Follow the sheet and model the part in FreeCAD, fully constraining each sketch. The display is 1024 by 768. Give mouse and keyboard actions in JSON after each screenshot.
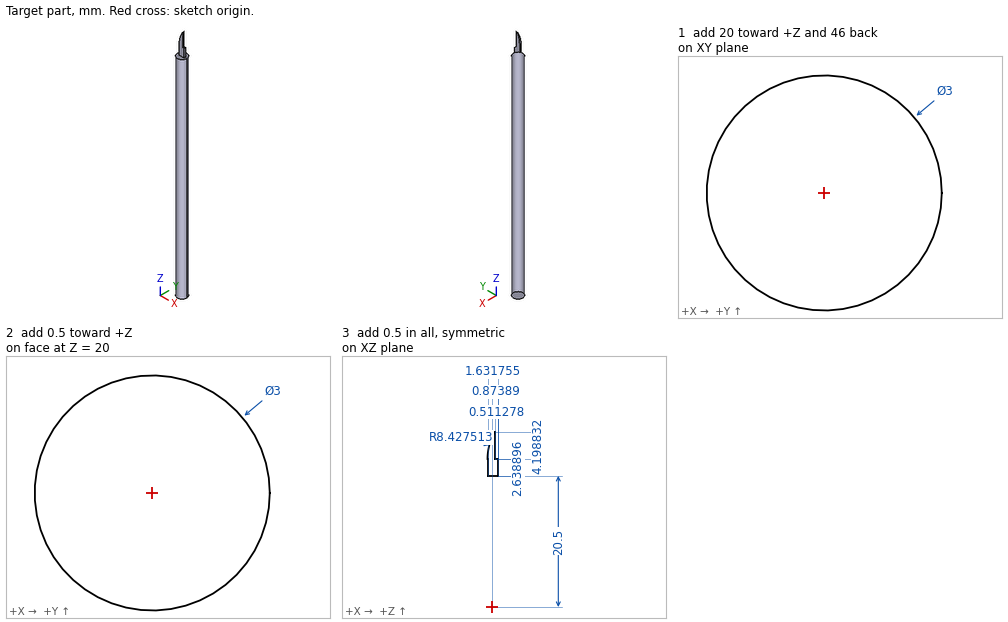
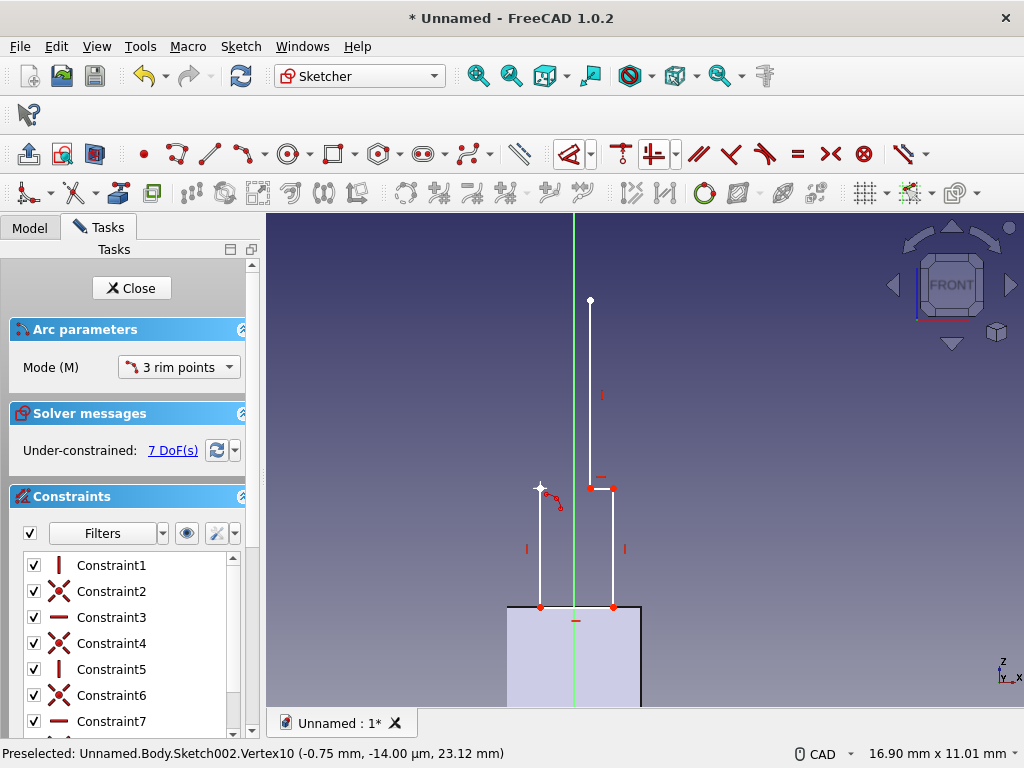
{"action": "left_click", "coordinate": [540, 489]}
{"action": "left_click", "coordinate": [590, 301]}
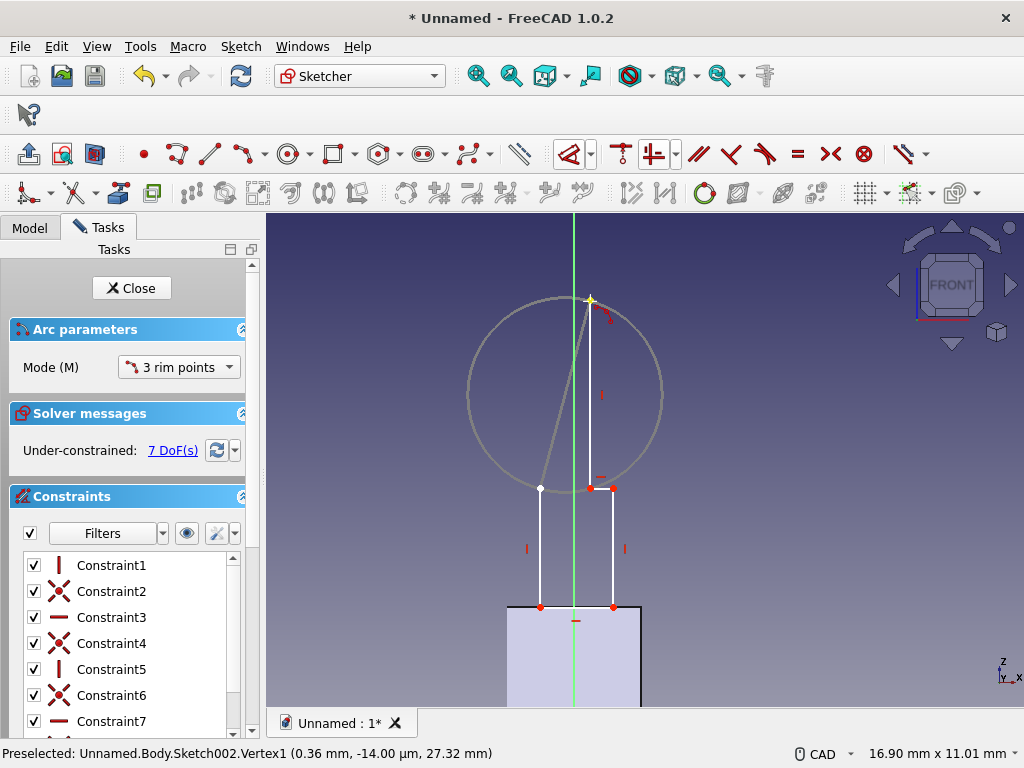
{"action": "scroll", "coordinate": [553, 391], "scroll_direction": "up", "scroll_amount": 2}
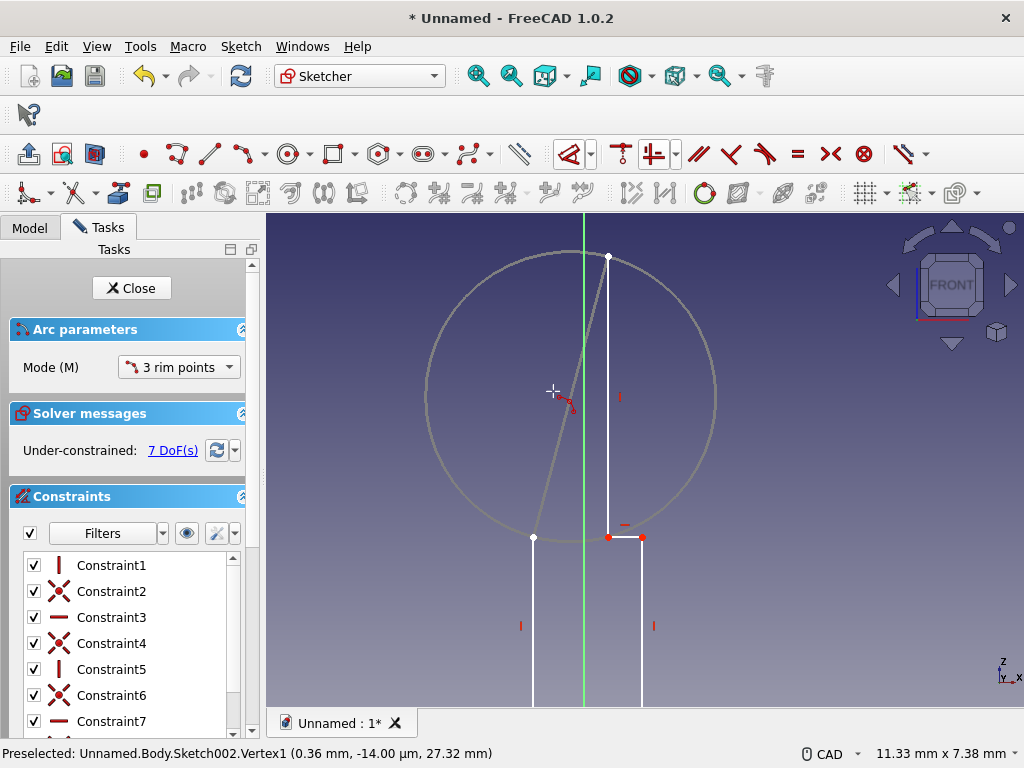
{"action": "left_click", "coordinate": [552, 391]}
{"action": "key", "text": "Escape"}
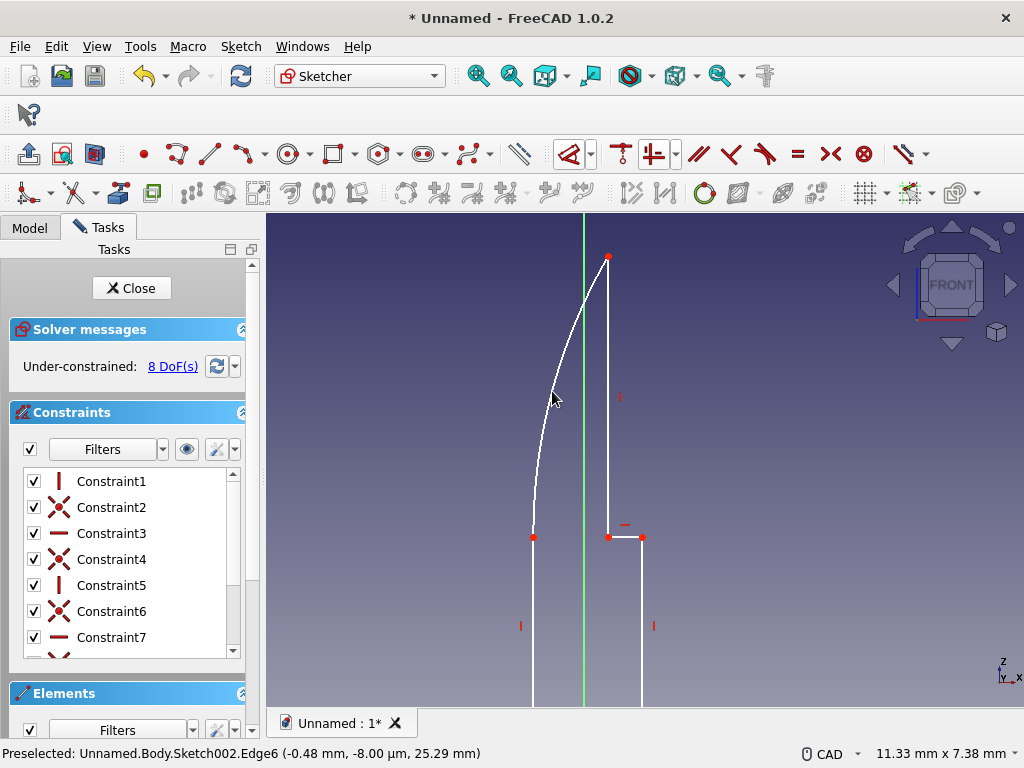
{"action": "left_click", "coordinate": [533, 661]}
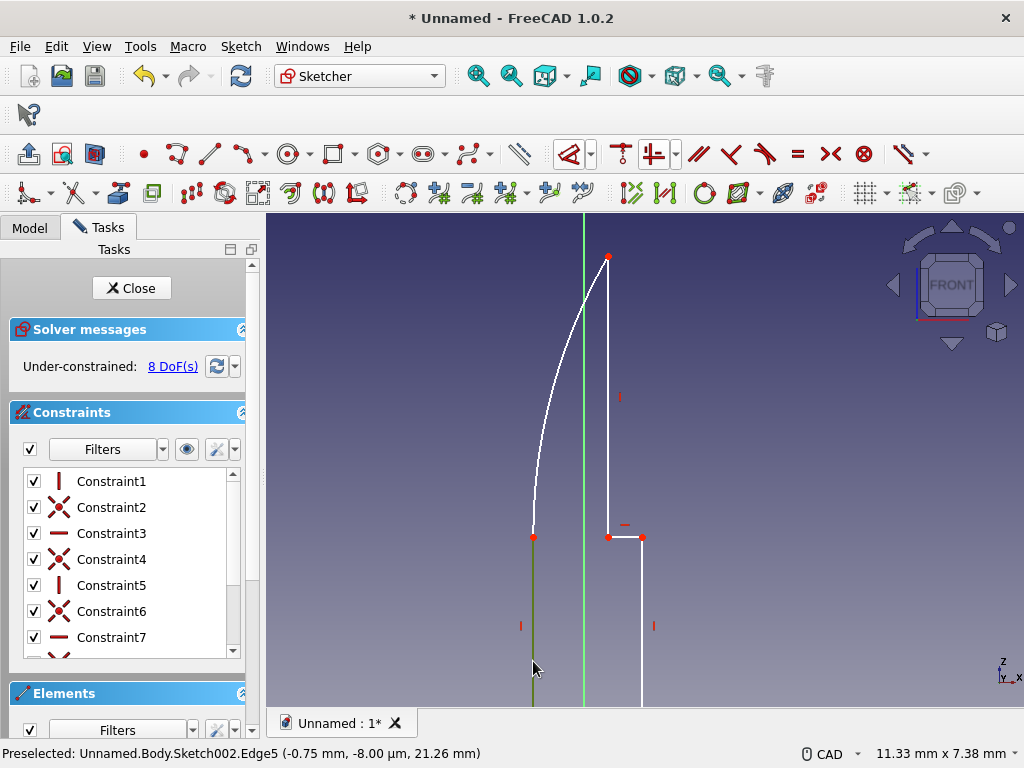
{"action": "left_click", "coordinate": [570, 336]}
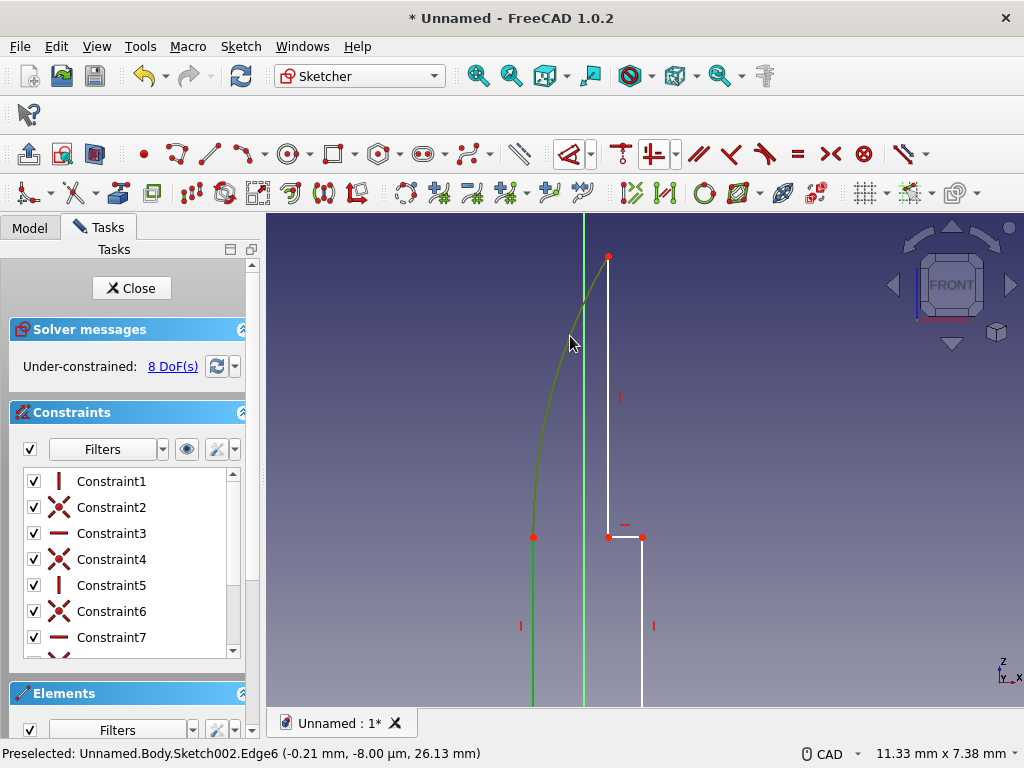
{"action": "left_click", "coordinate": [765, 154]}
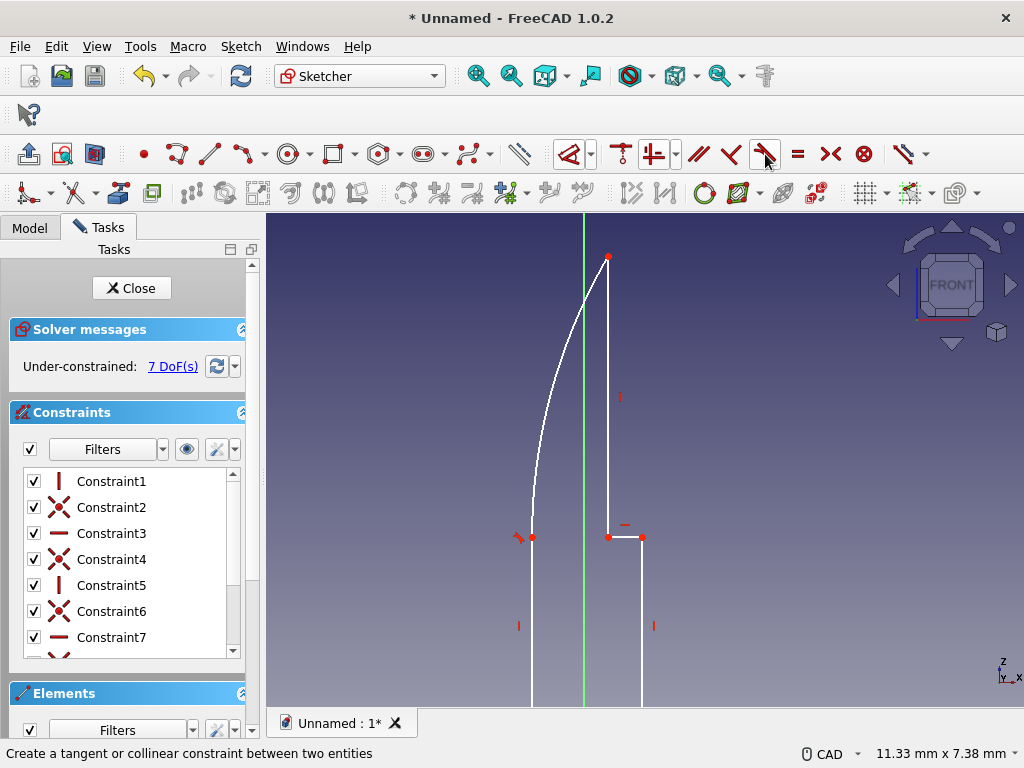
{"action": "left_click", "coordinate": [568, 154]}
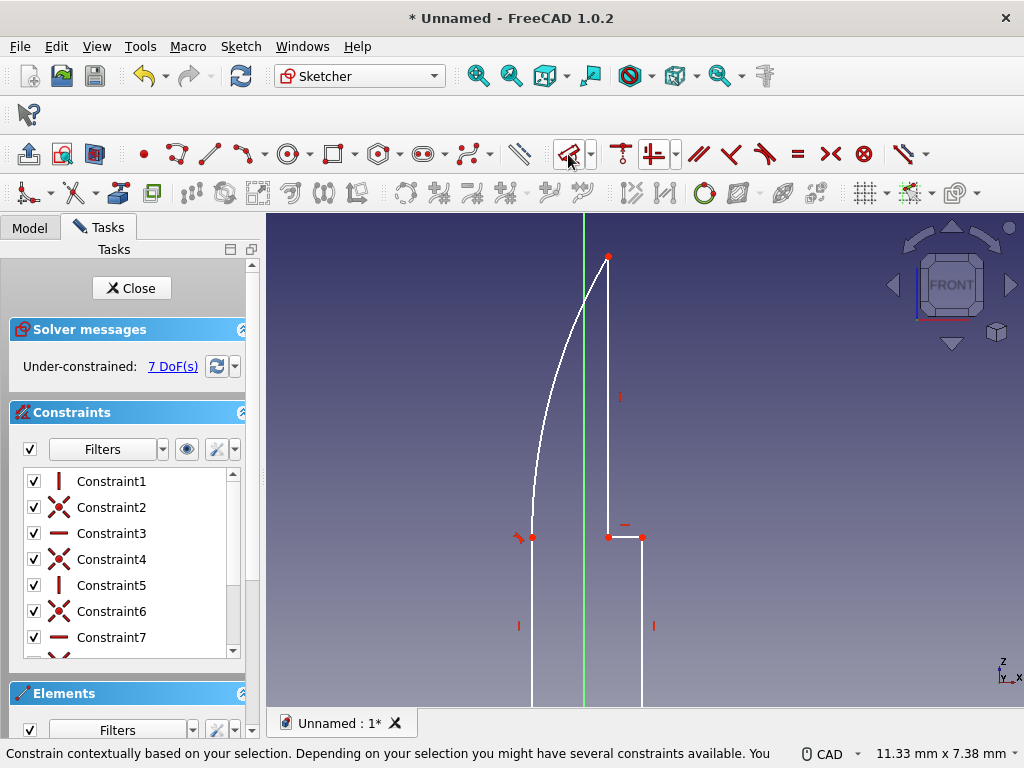
{"action": "left_click", "coordinate": [570, 336]}
{"action": "left_click", "coordinate": [540, 324]}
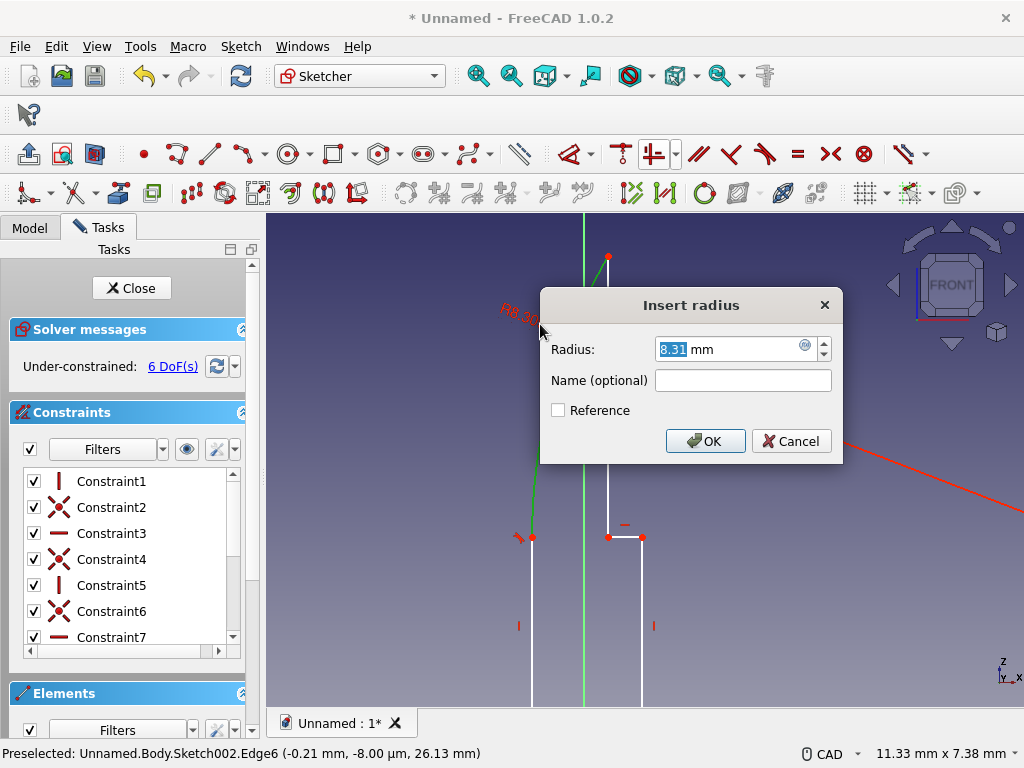
{"action": "type", "text": "8.427513"}
{"action": "key", "text": "Return"}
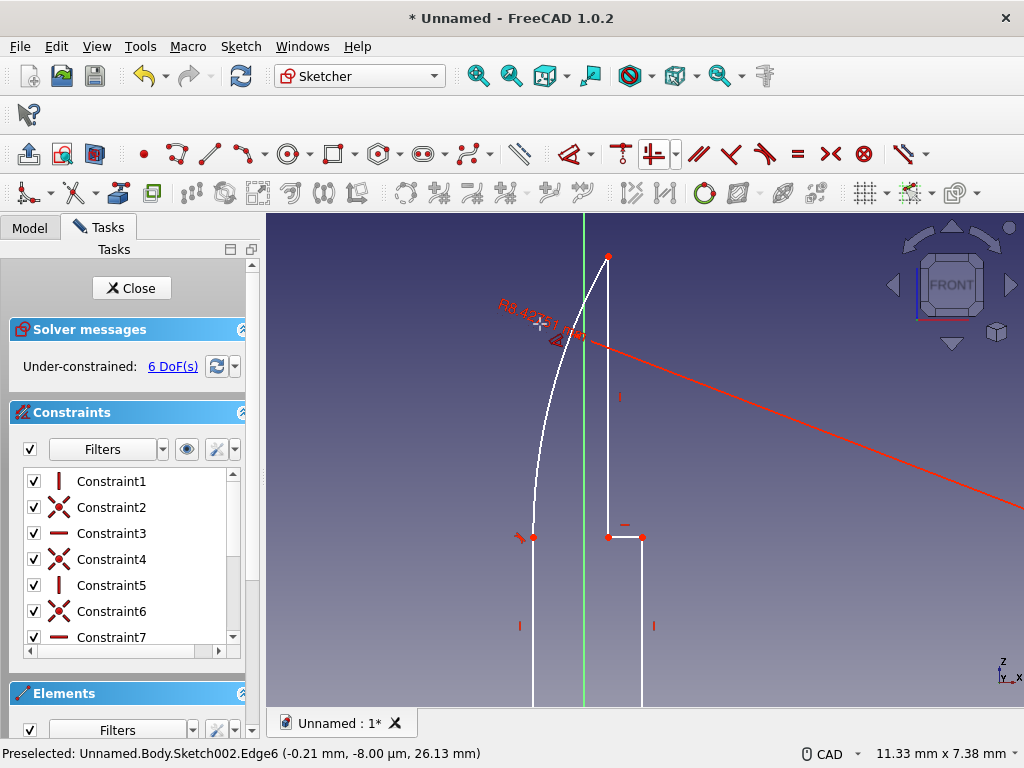
{"action": "scroll", "coordinate": [554, 412], "scroll_direction": "down", "scroll_amount": 2}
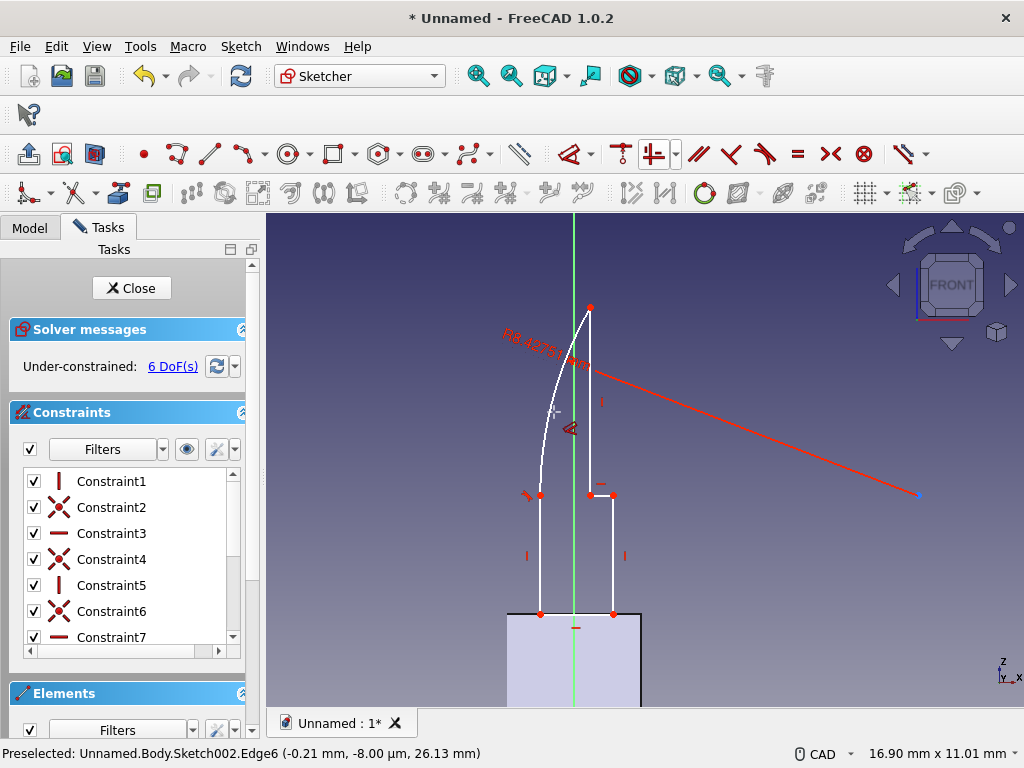
{"action": "left_click", "coordinate": [613, 615]}
{"action": "left_click", "coordinate": [647, 647]}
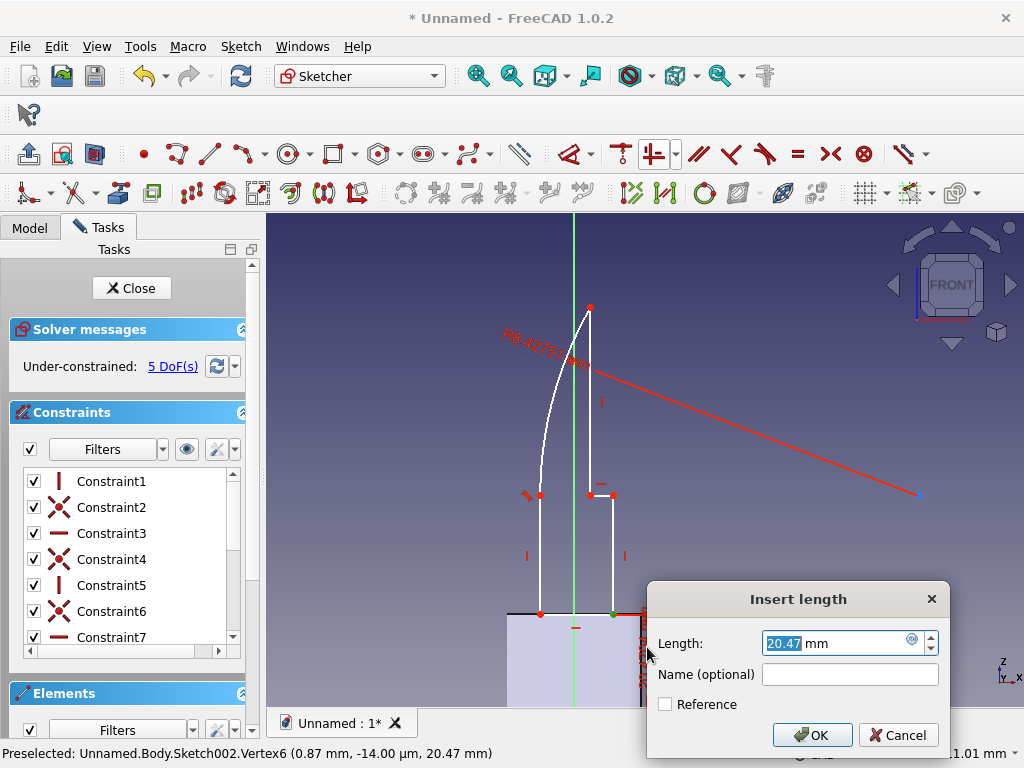
{"action": "type", "text": "20.5"}
{"action": "key", "text": "Return"}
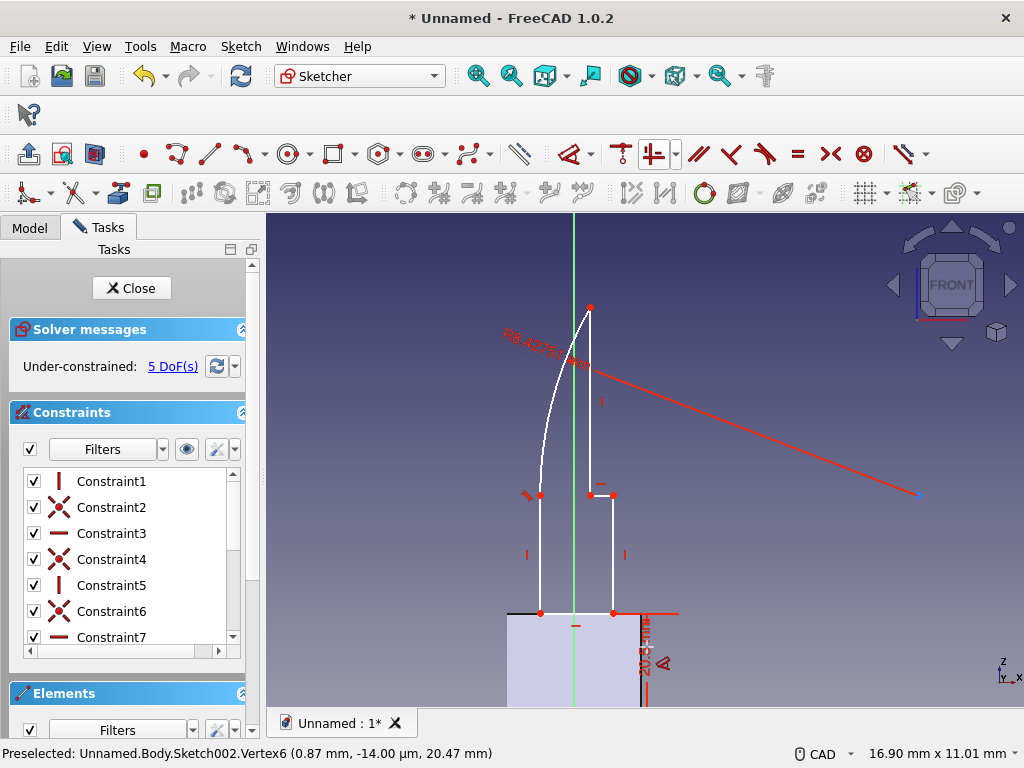
{"action": "left_click", "coordinate": [590, 364]}
{"action": "left_click", "coordinate": [624, 402]}